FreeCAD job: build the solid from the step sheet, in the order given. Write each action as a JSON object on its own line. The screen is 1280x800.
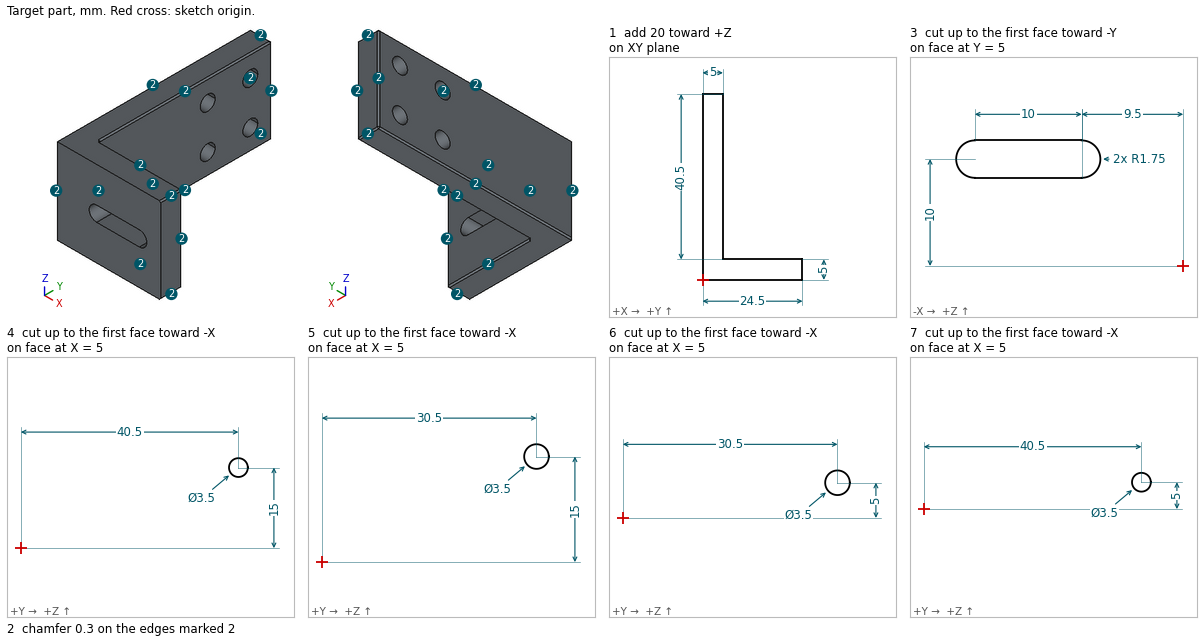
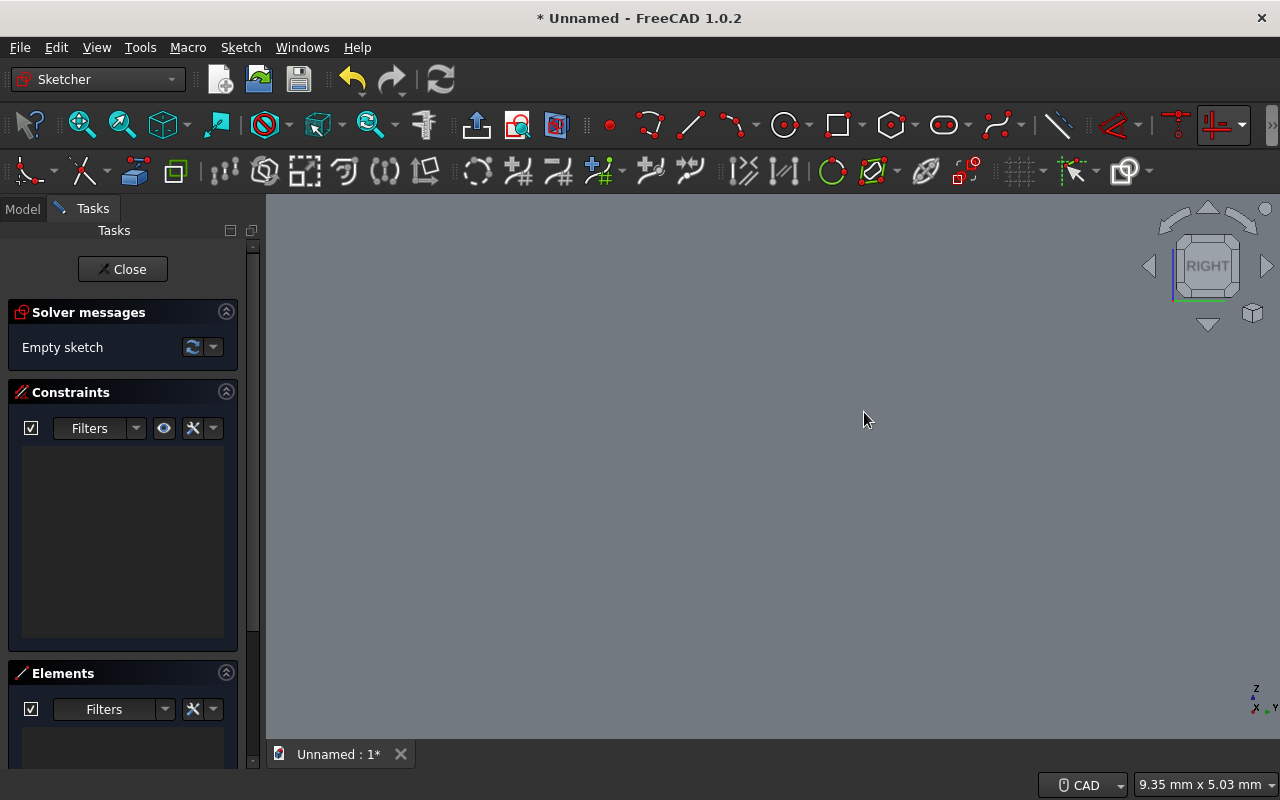
{"action": "left_click", "coordinate": [786, 126]}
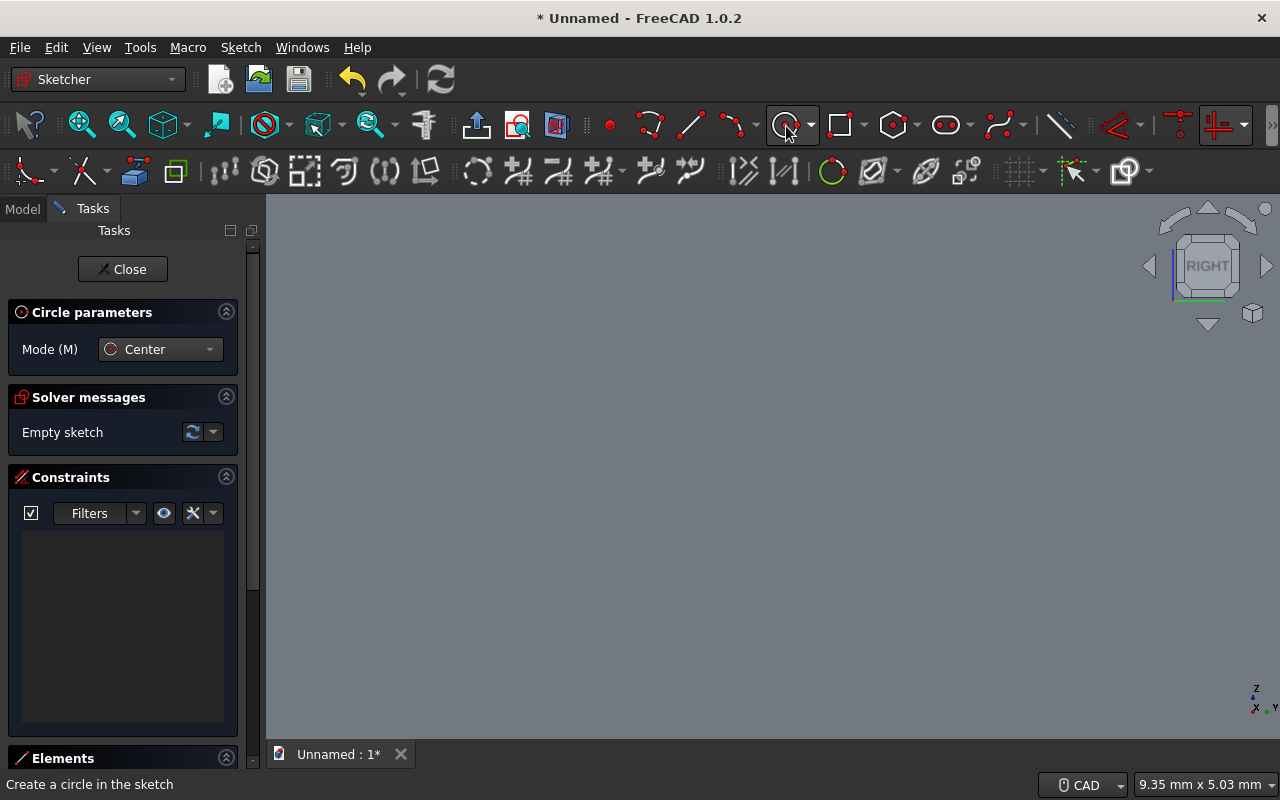
{"action": "left_click", "coordinate": [695, 467]}
{"action": "left_click", "coordinate": [829, 333]}
{"action": "key", "text": "Escape"}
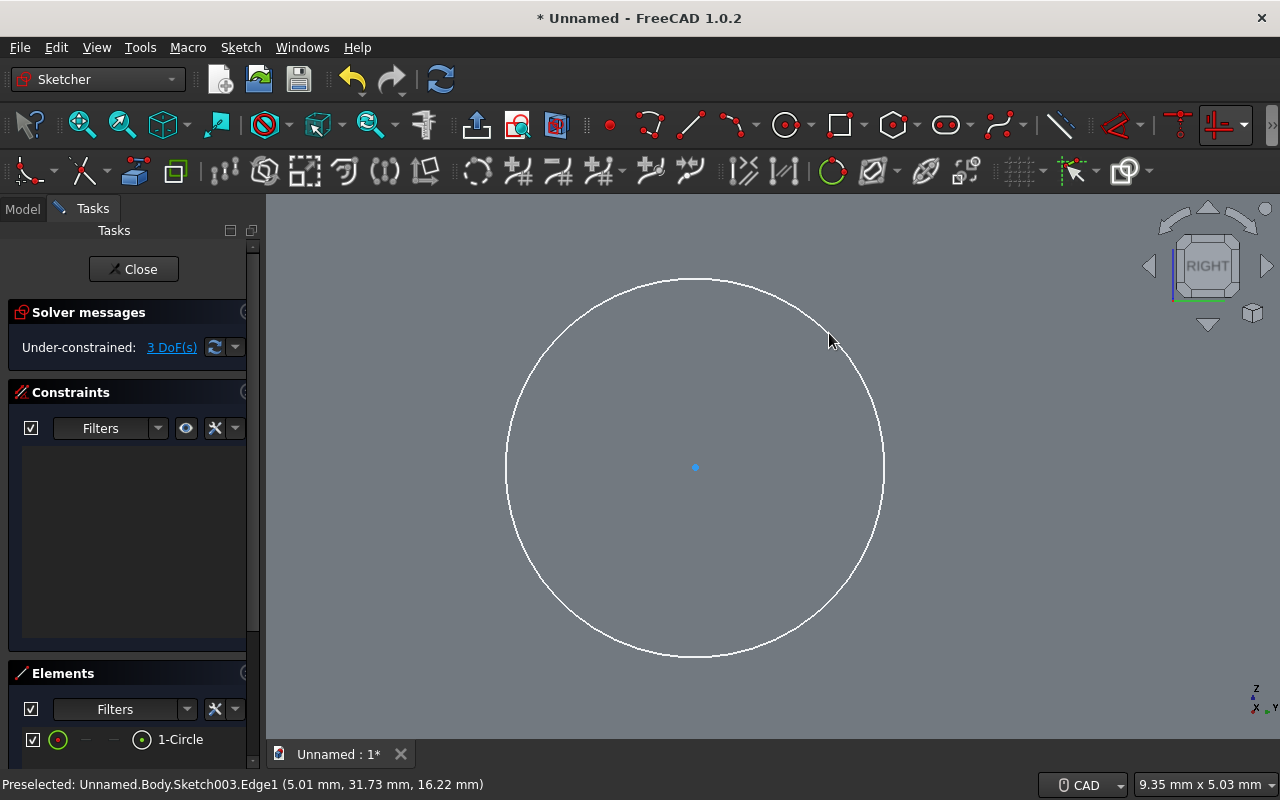
{"action": "key", "text": "d"}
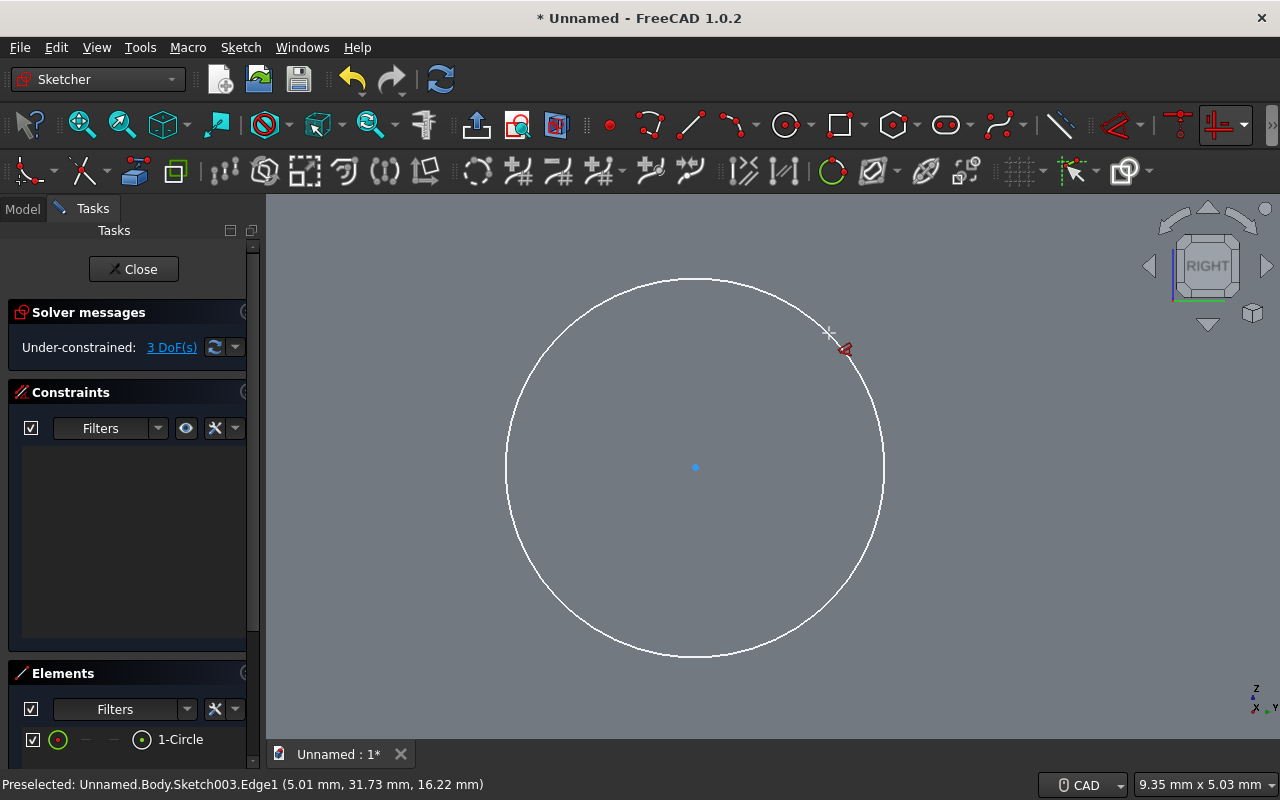
{"action": "left_click", "coordinate": [829, 334]}
{"action": "left_click", "coordinate": [852, 311]}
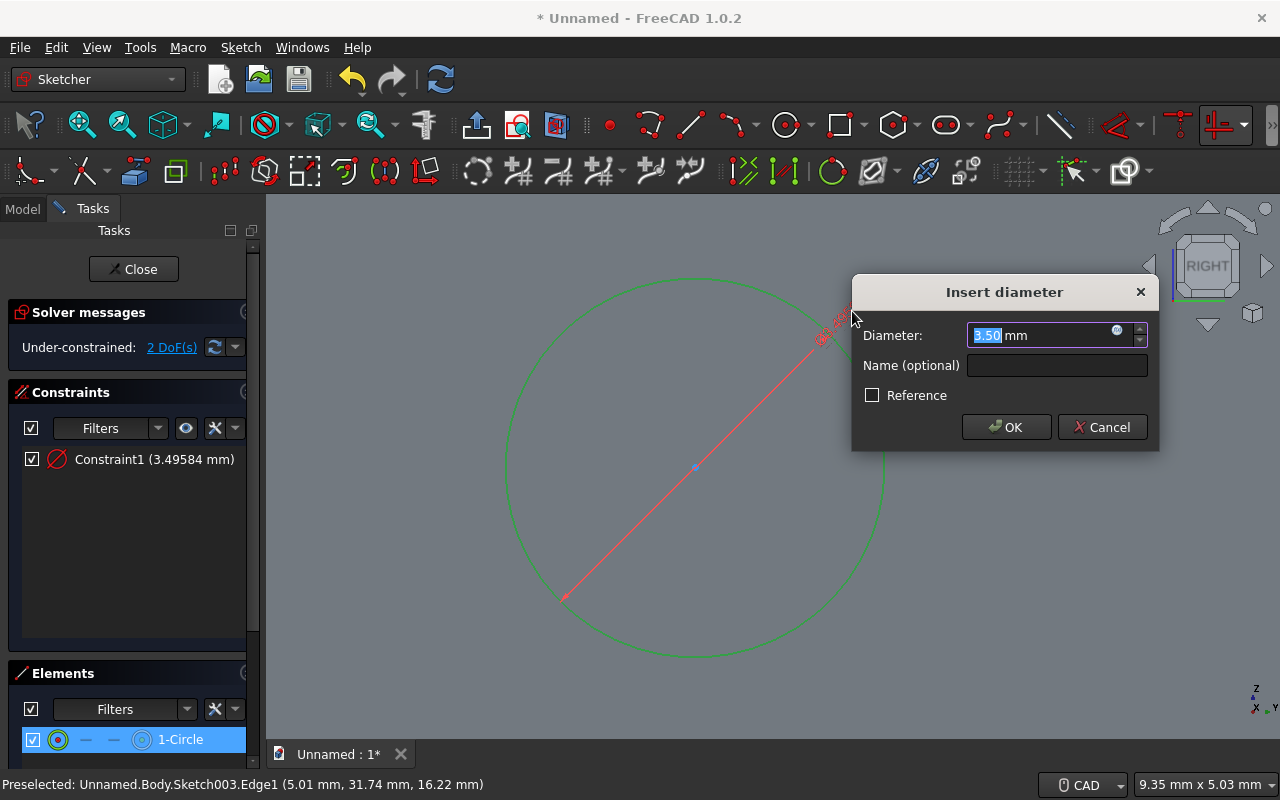
{"action": "type", "text": "3.5"}
{"action": "key", "text": "Return"}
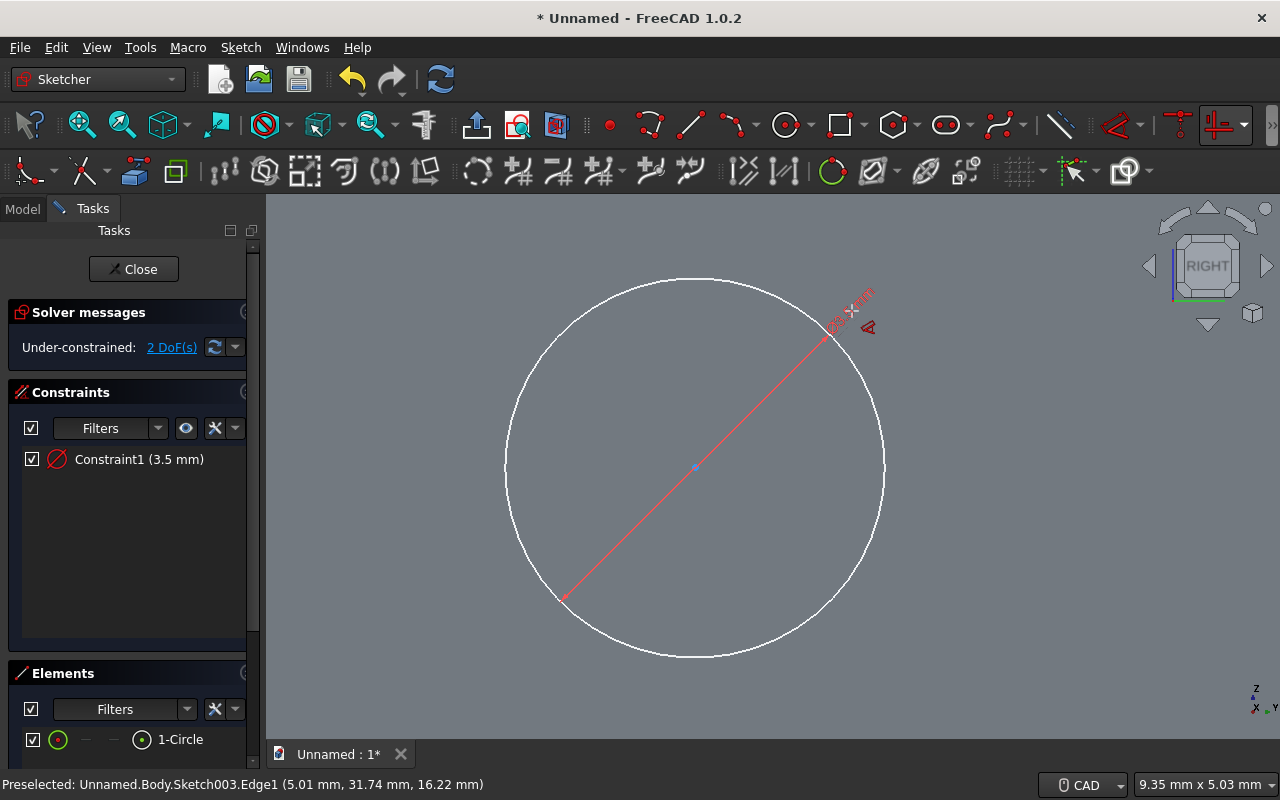
{"action": "left_click", "coordinate": [695, 468]}
{"action": "left_click", "coordinate": [729, 589]}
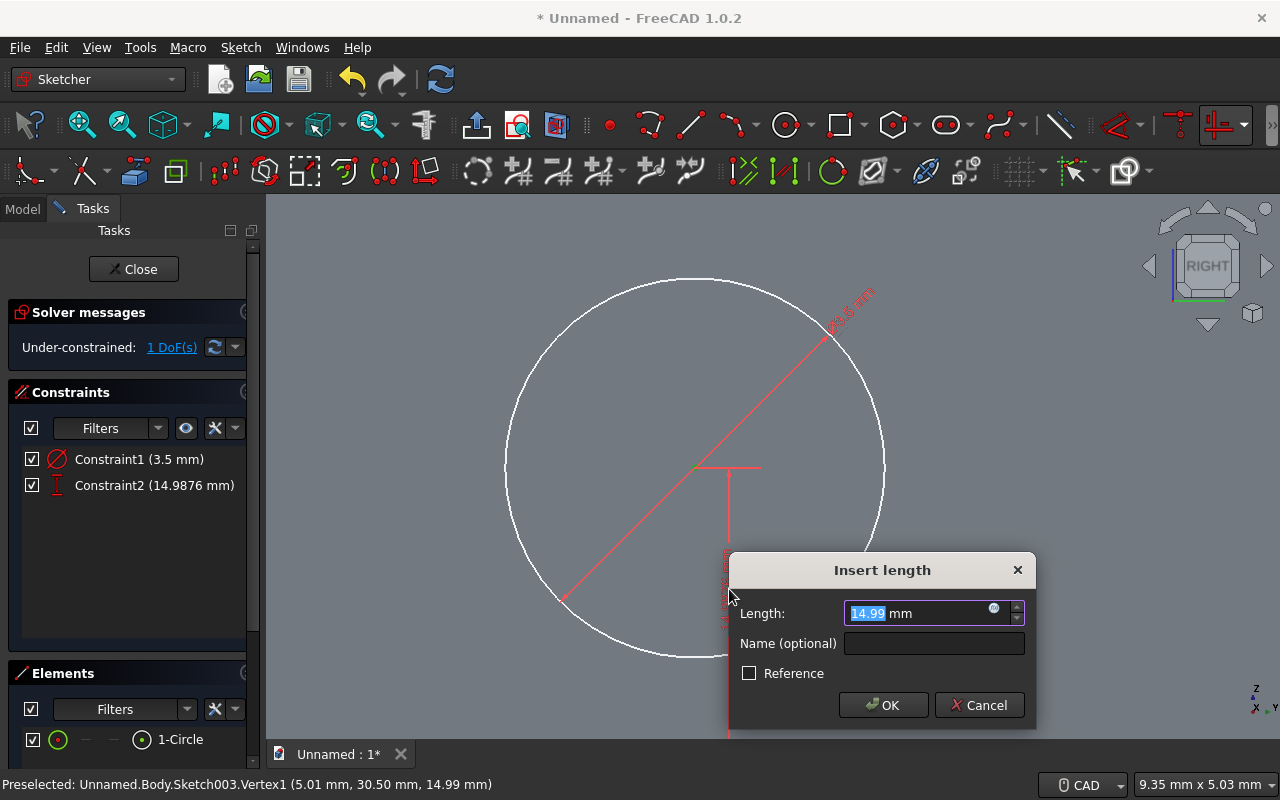
{"action": "type", "text": "15"}
{"action": "key", "text": "Return"}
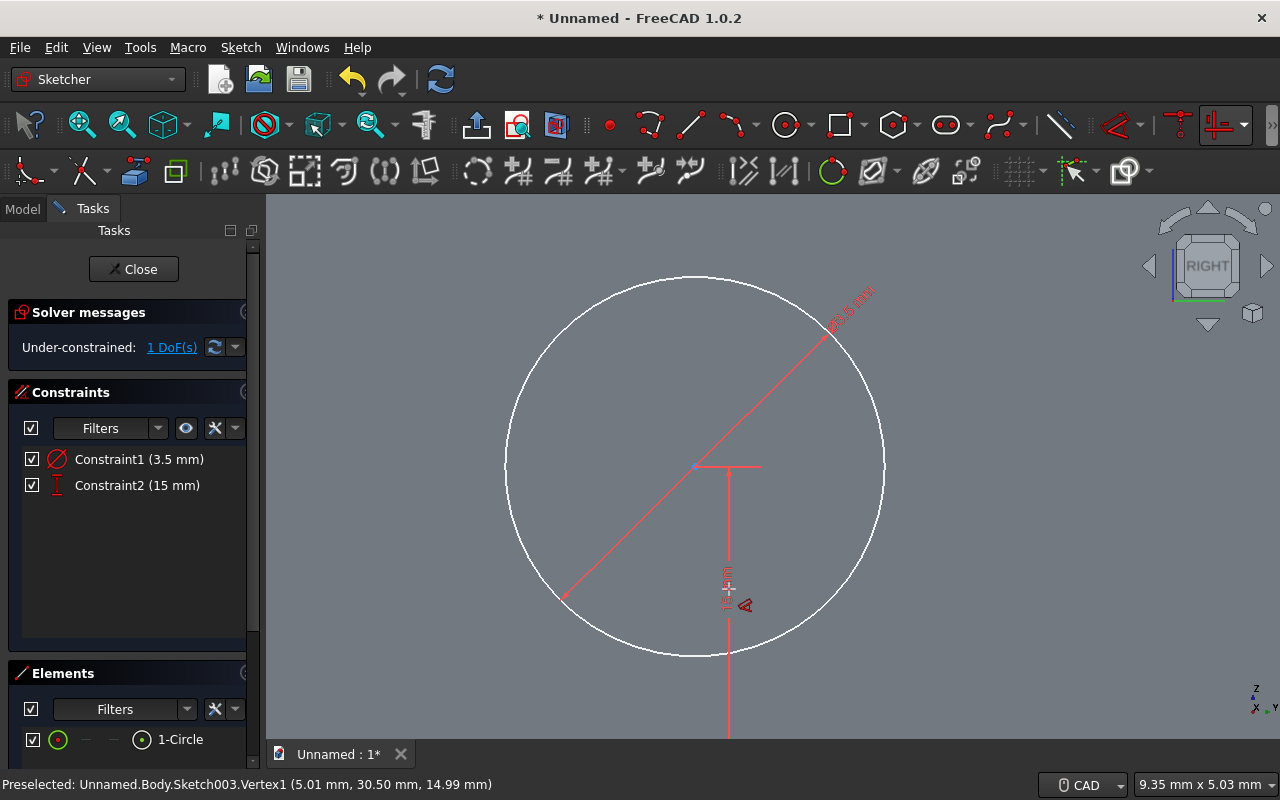
{"action": "left_click", "coordinate": [695, 467]}
{"action": "left_click", "coordinate": [494, 433]}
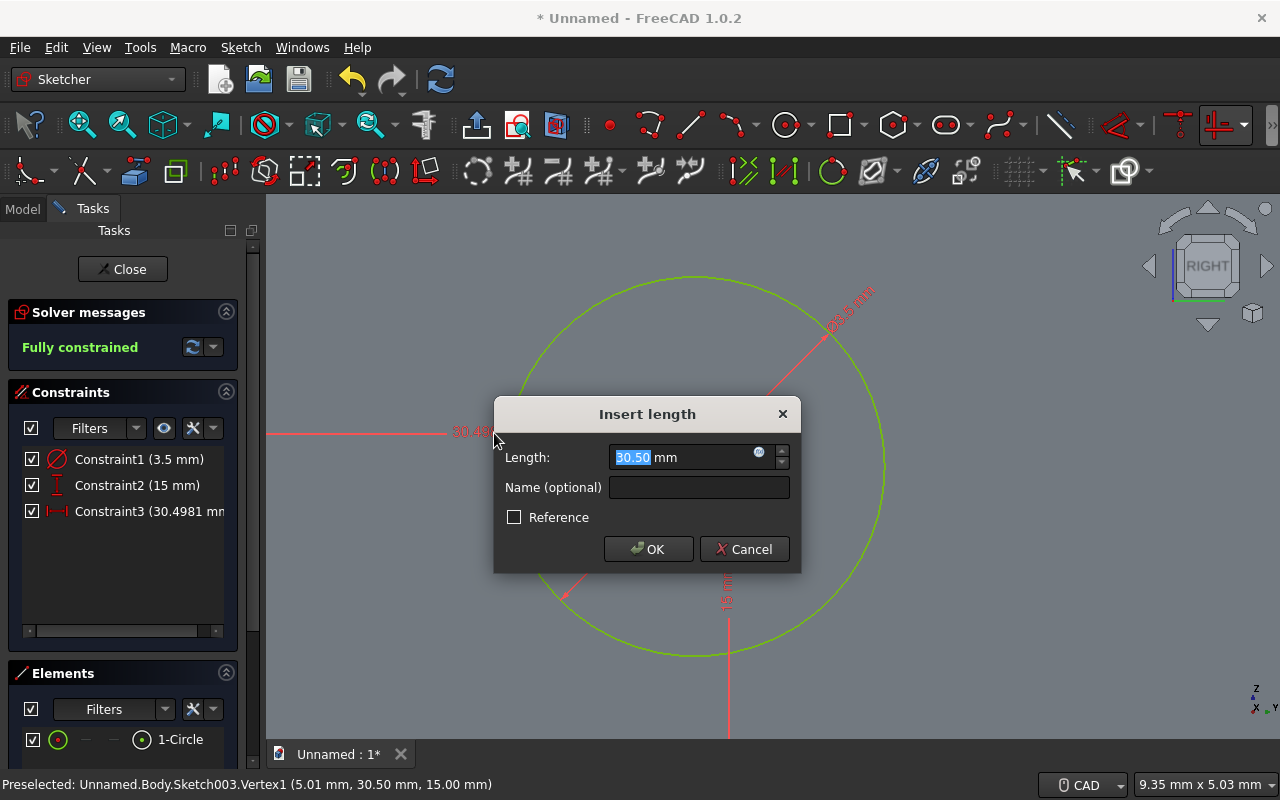
{"action": "type", "text": "30.5"}
{"action": "key", "text": "Return"}
{"action": "key", "text": "Escape"}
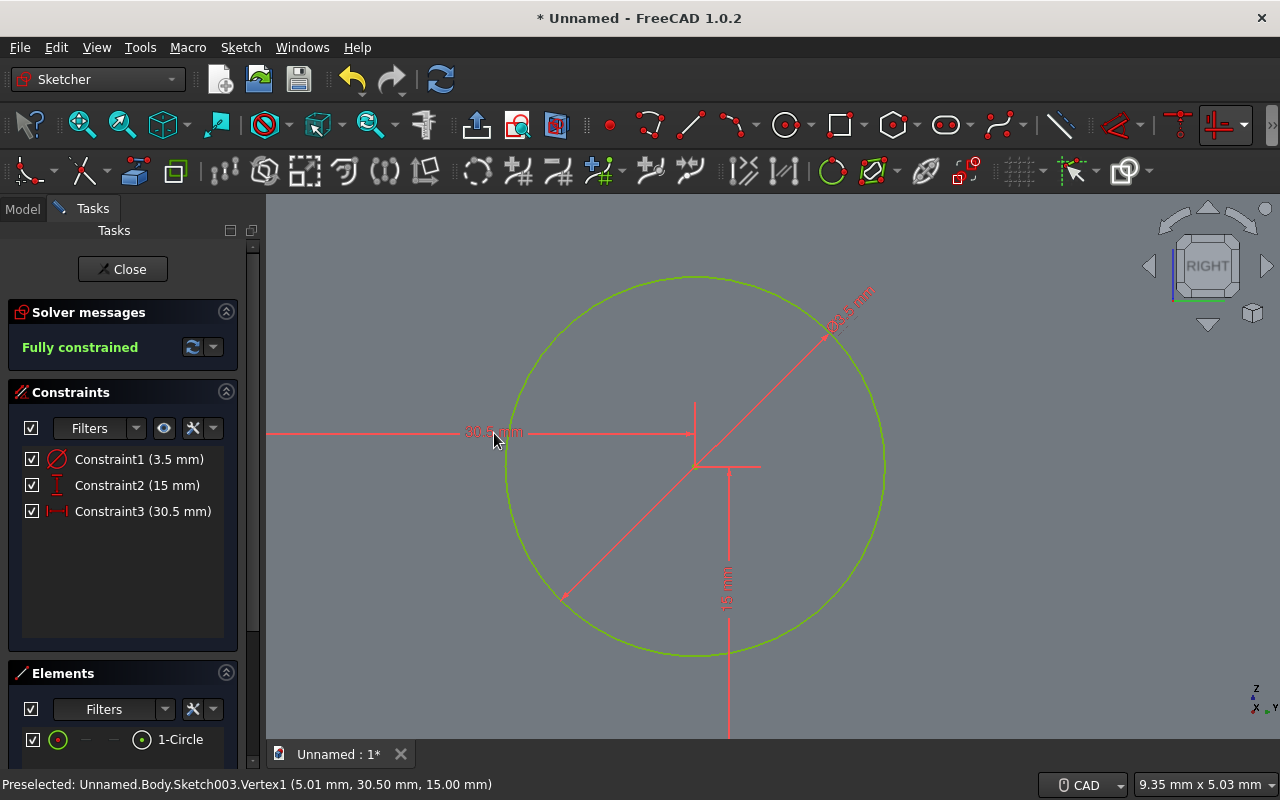
{"action": "left_click", "coordinate": [123, 269]}